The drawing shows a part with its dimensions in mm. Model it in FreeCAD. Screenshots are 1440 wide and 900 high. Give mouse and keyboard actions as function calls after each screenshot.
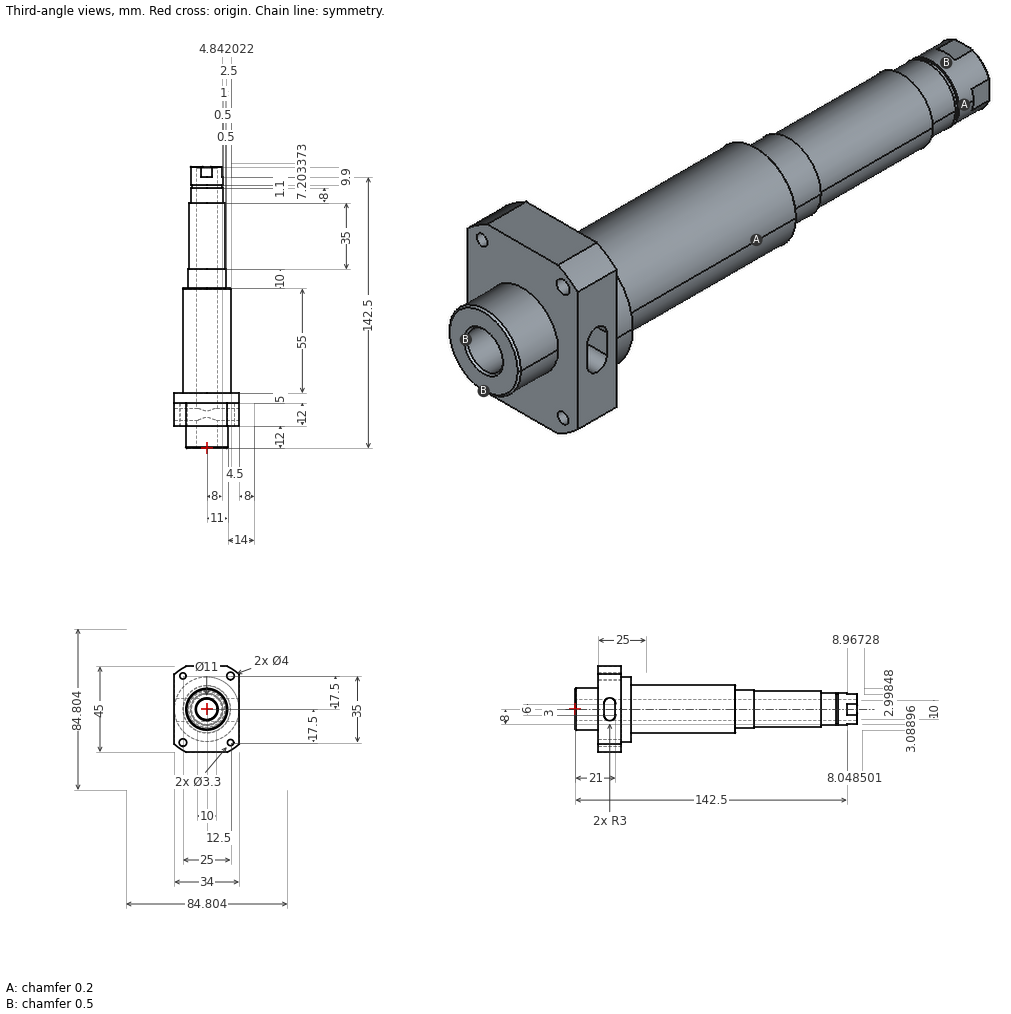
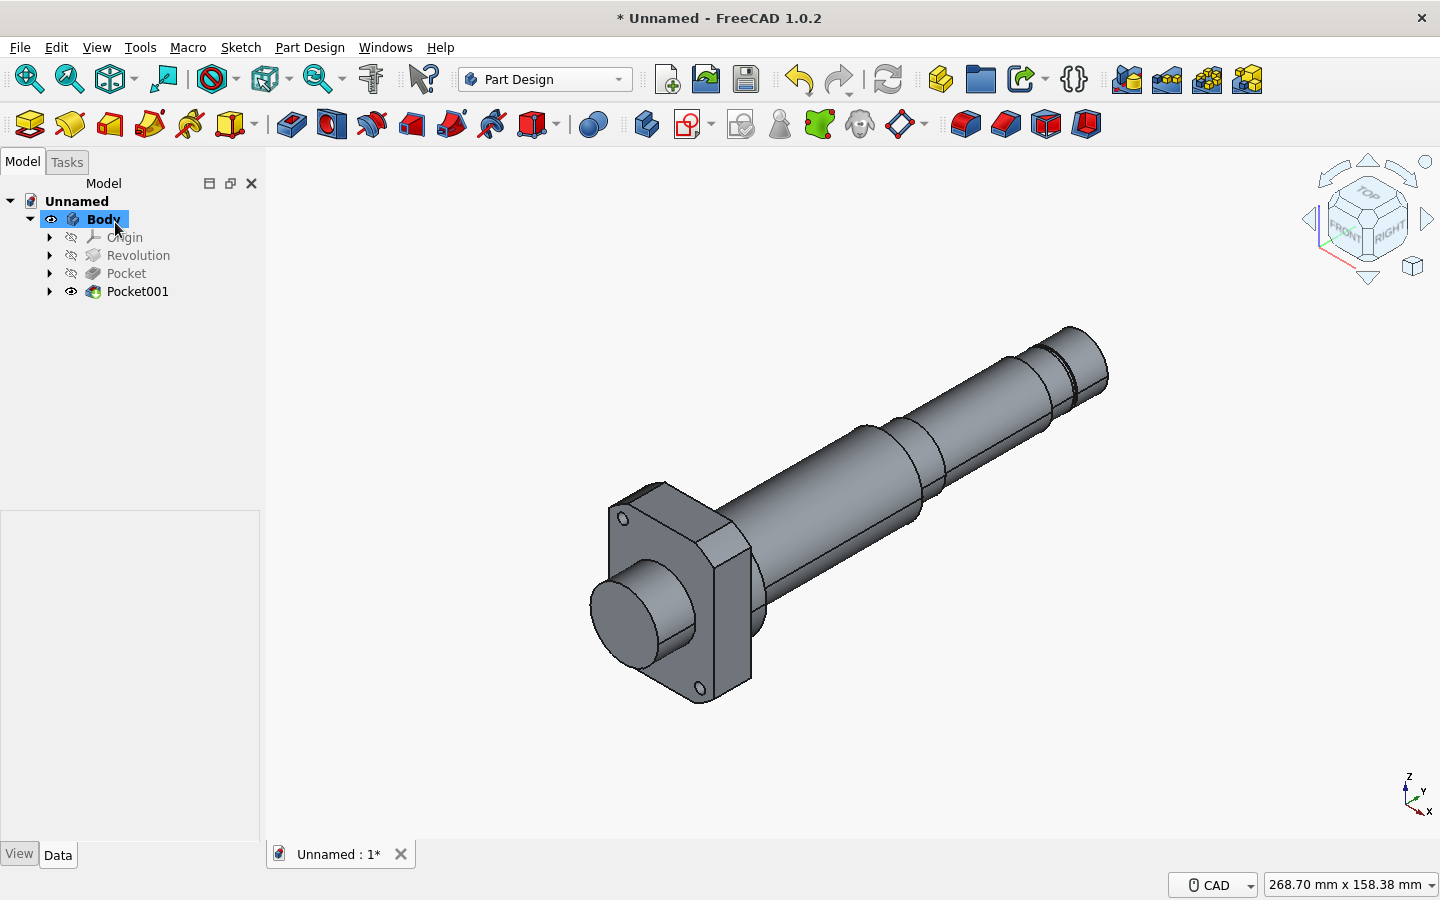
click(691, 574)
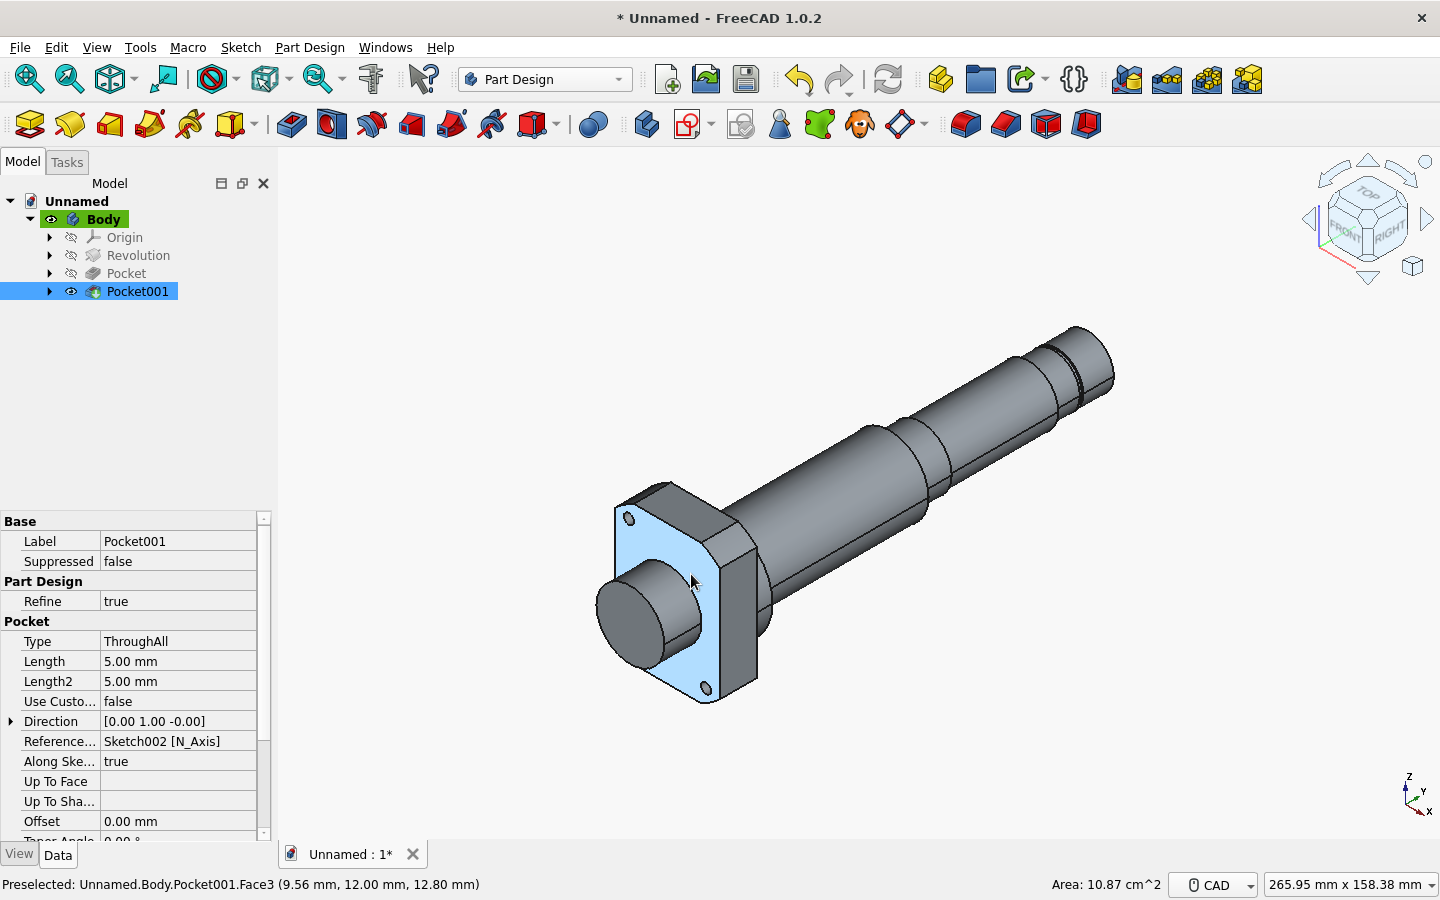
click(688, 124)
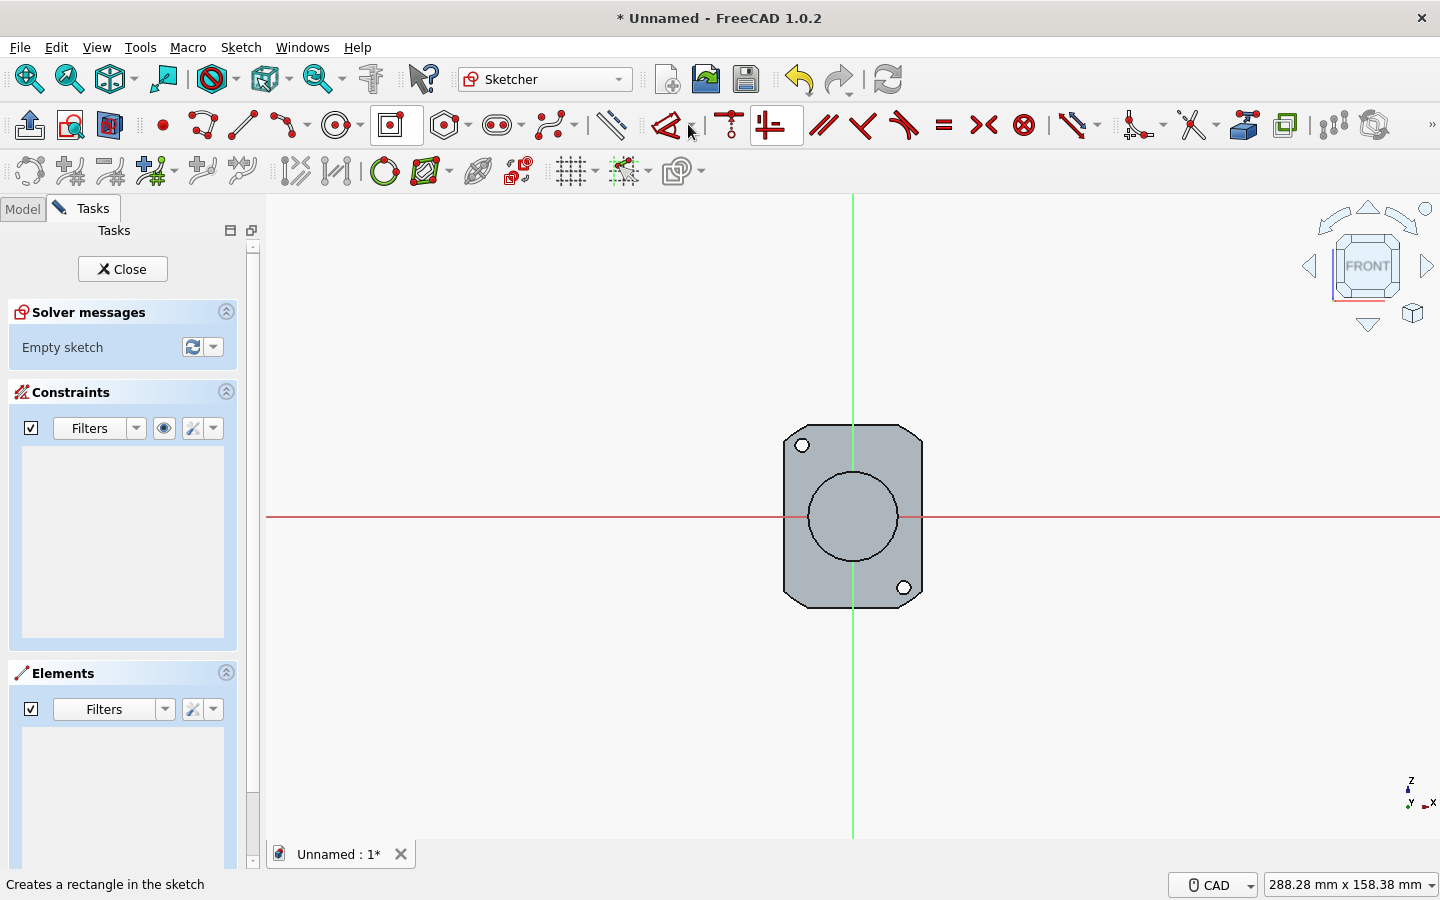
key(q)
key(s)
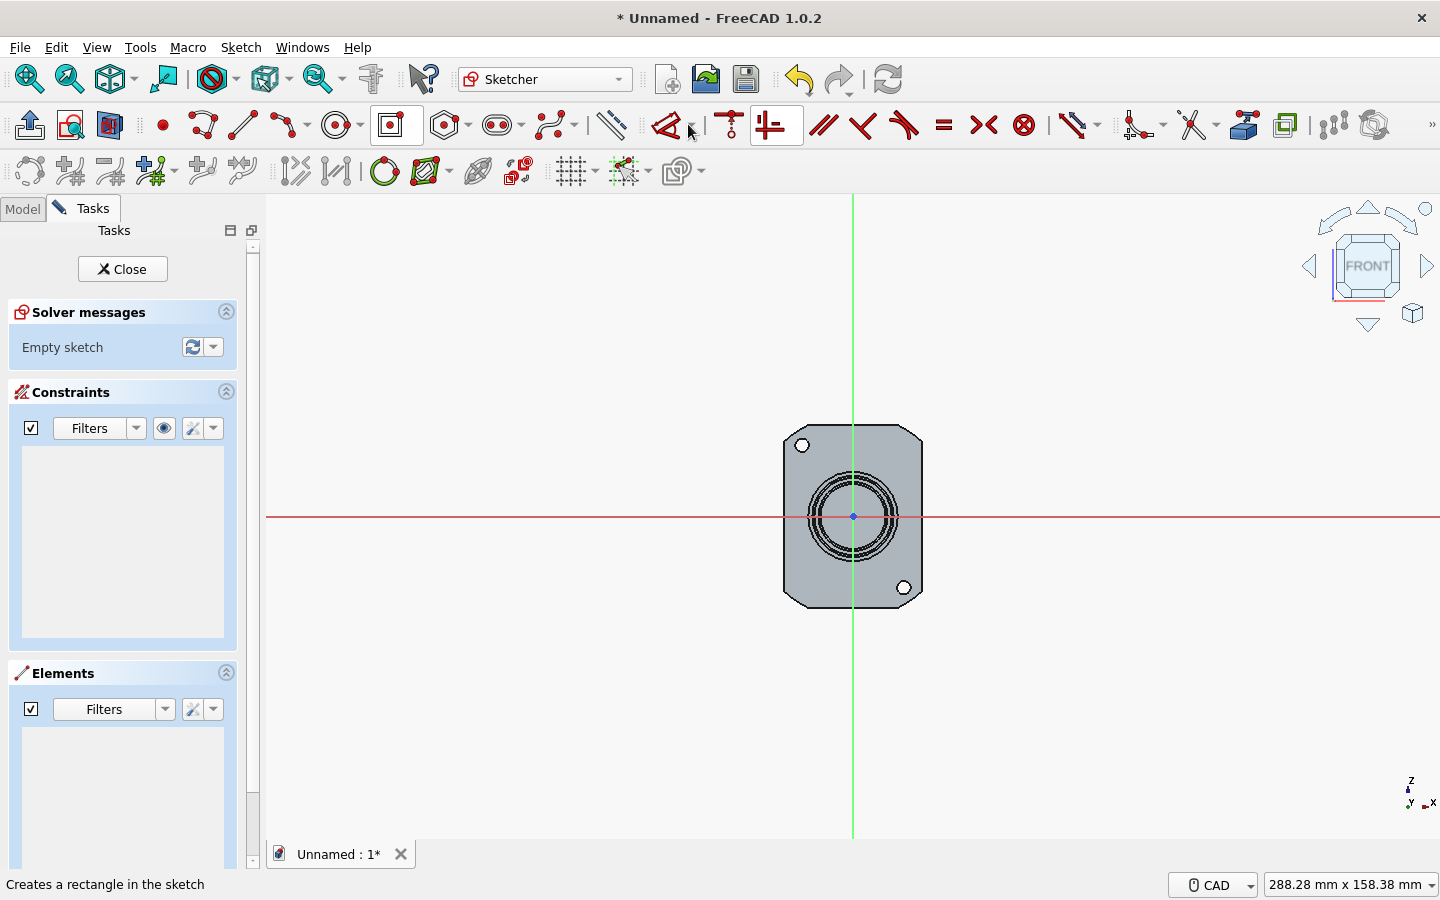
scroll(893, 516, up, 5)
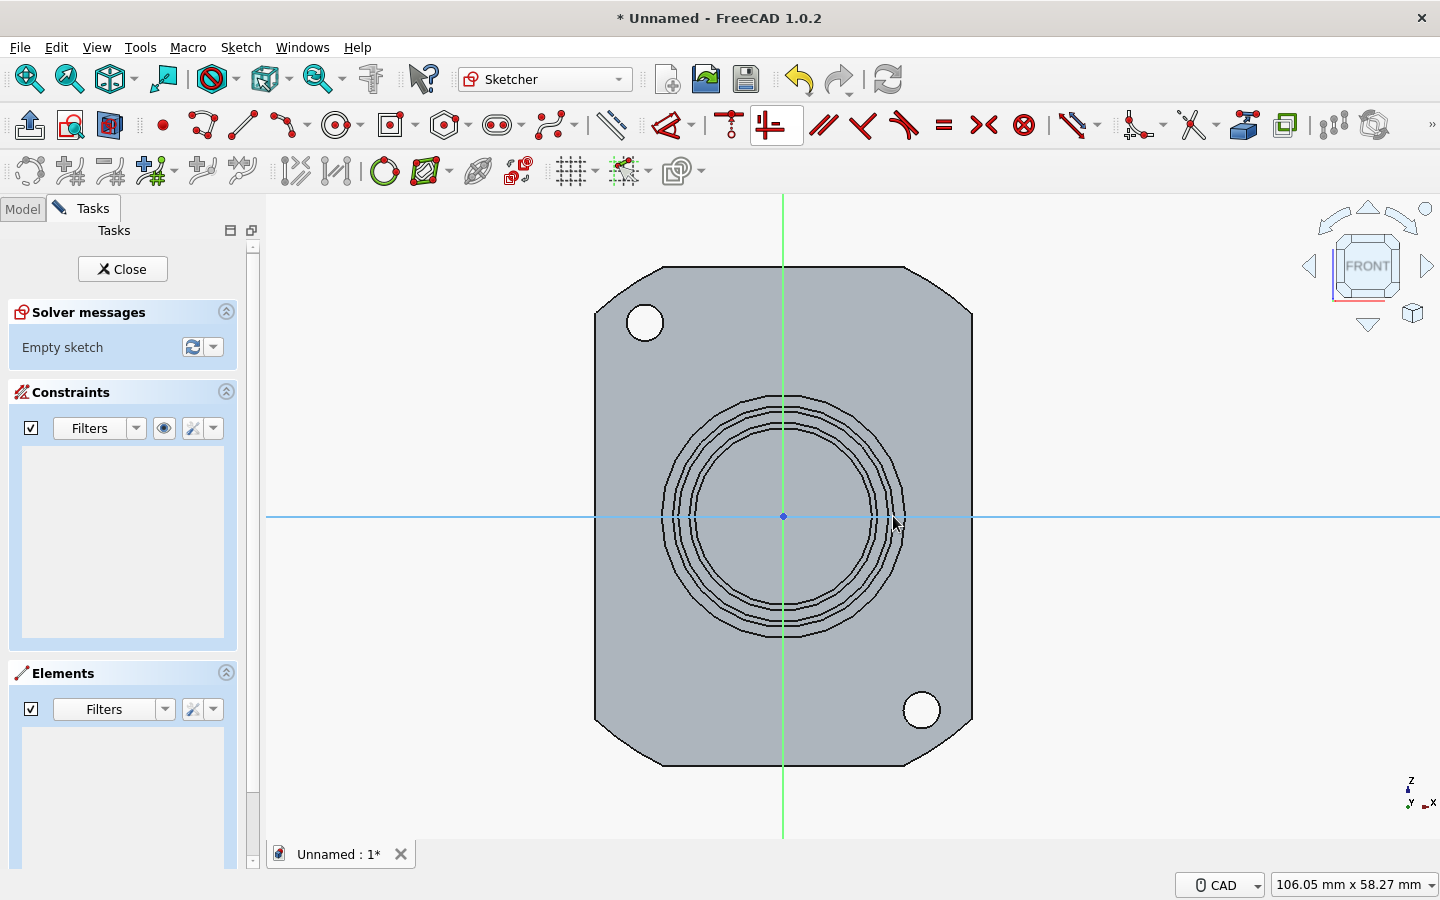
key(g)
key(c)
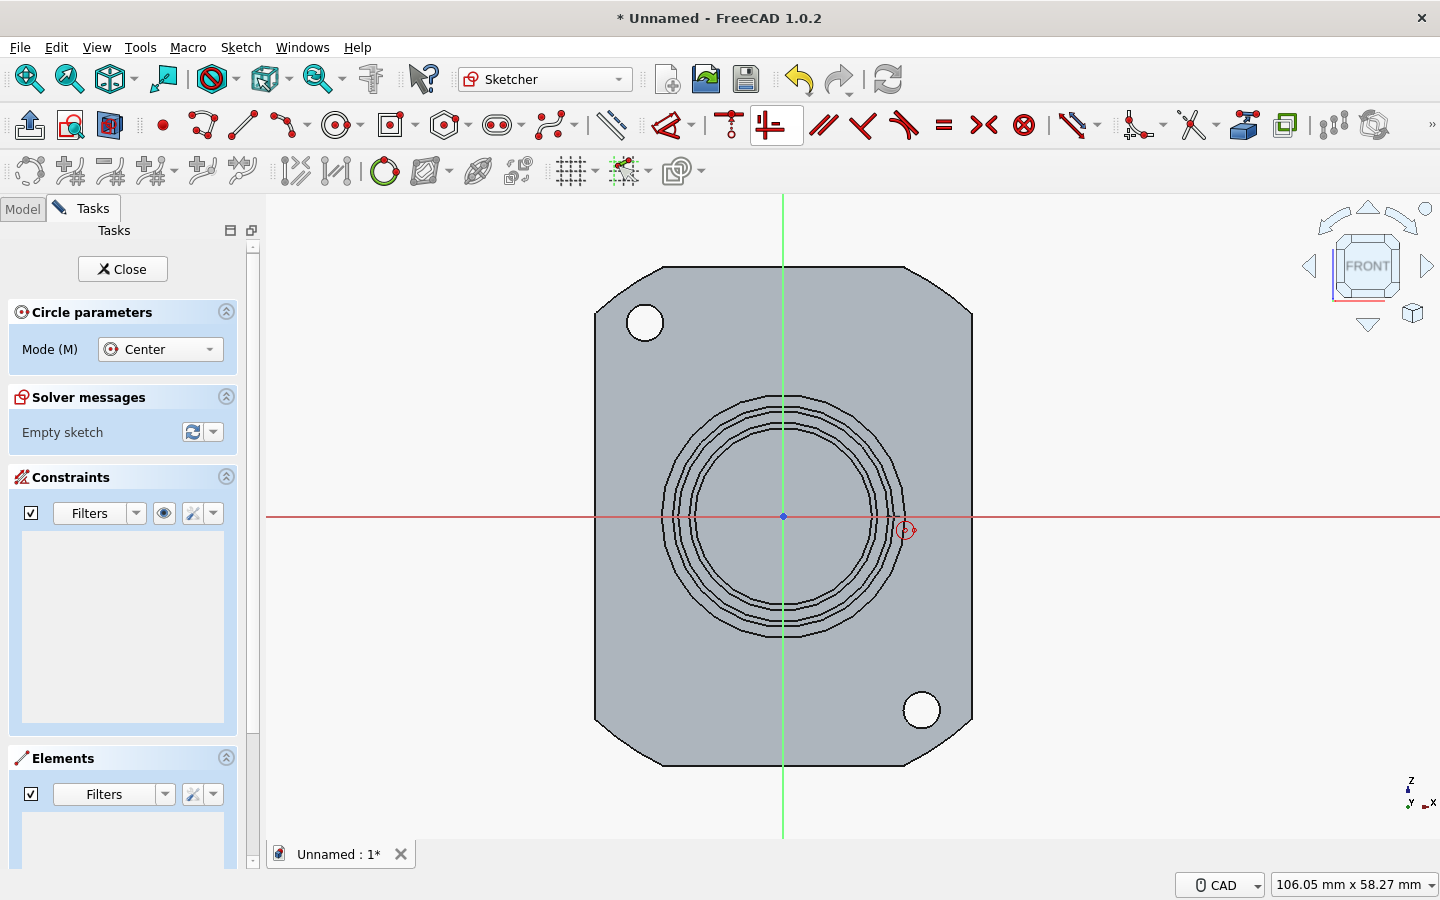
click(922, 323)
move(937, 307)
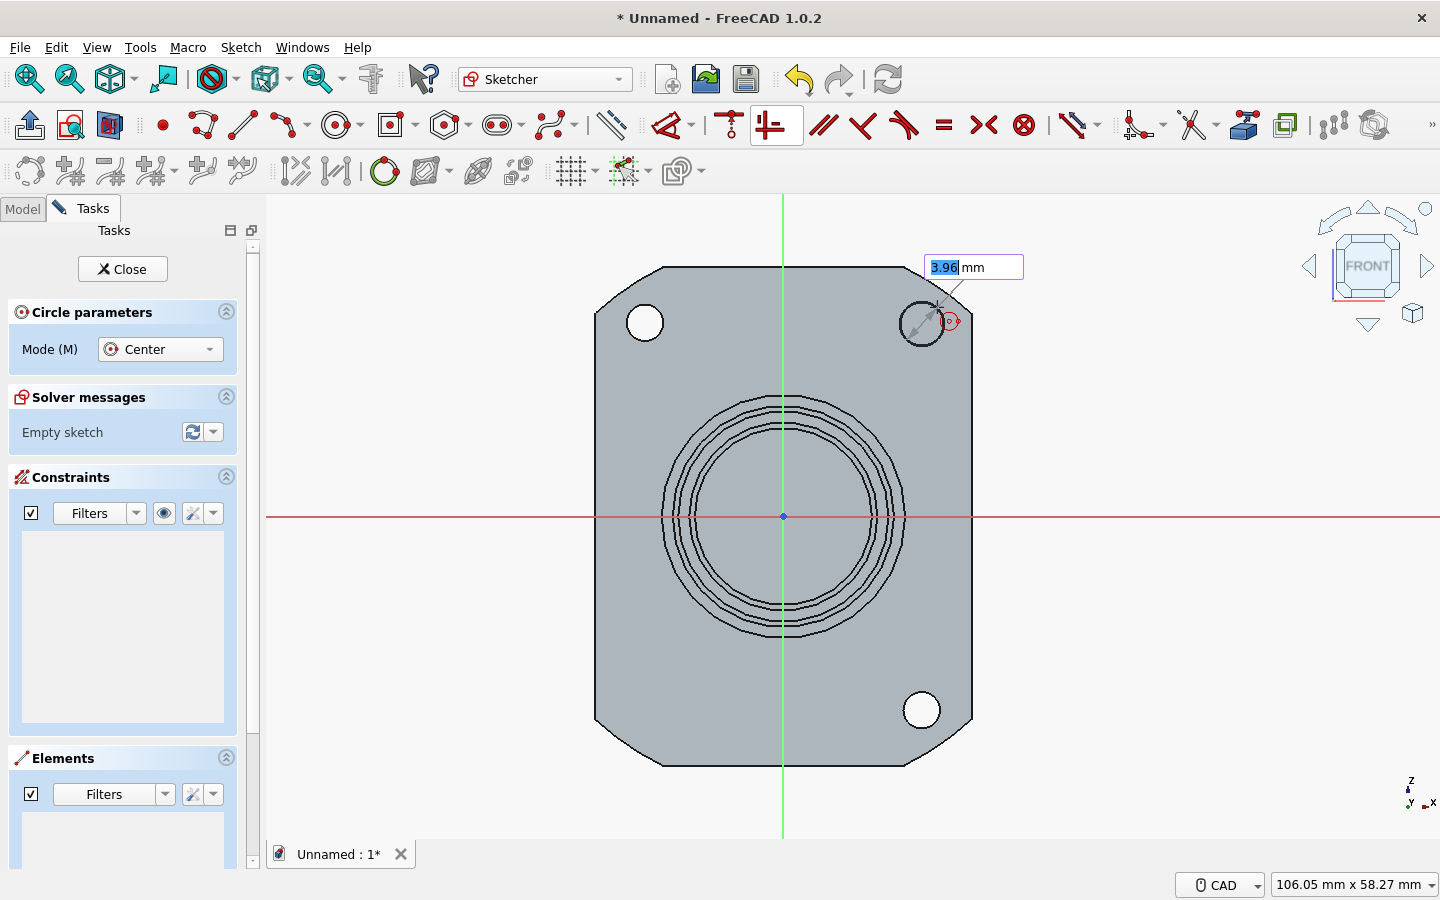
text(4)
key(Return)